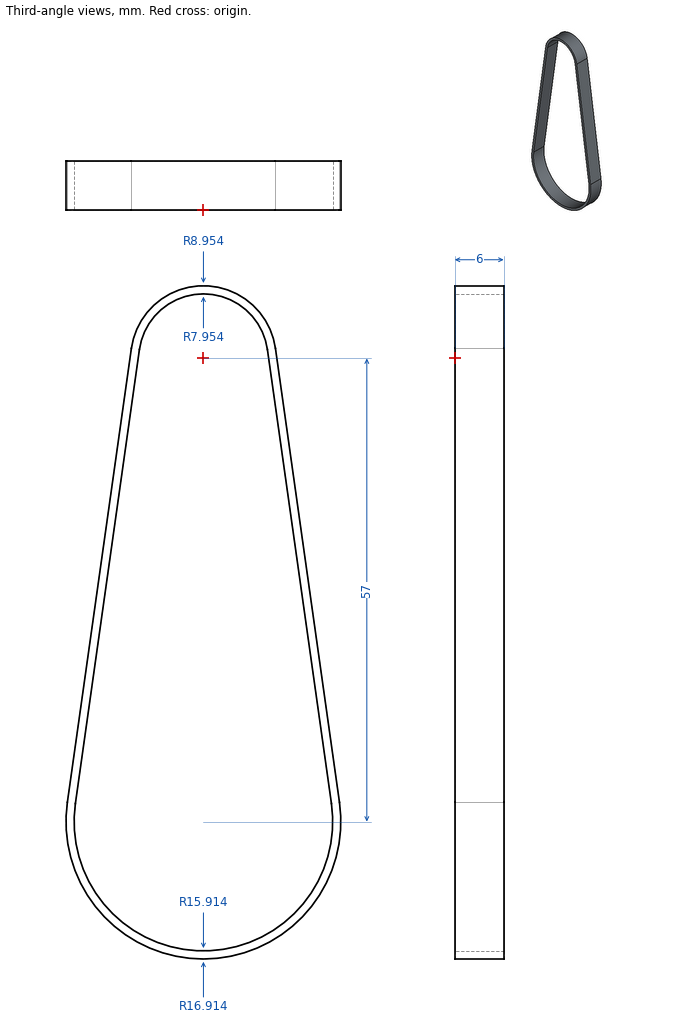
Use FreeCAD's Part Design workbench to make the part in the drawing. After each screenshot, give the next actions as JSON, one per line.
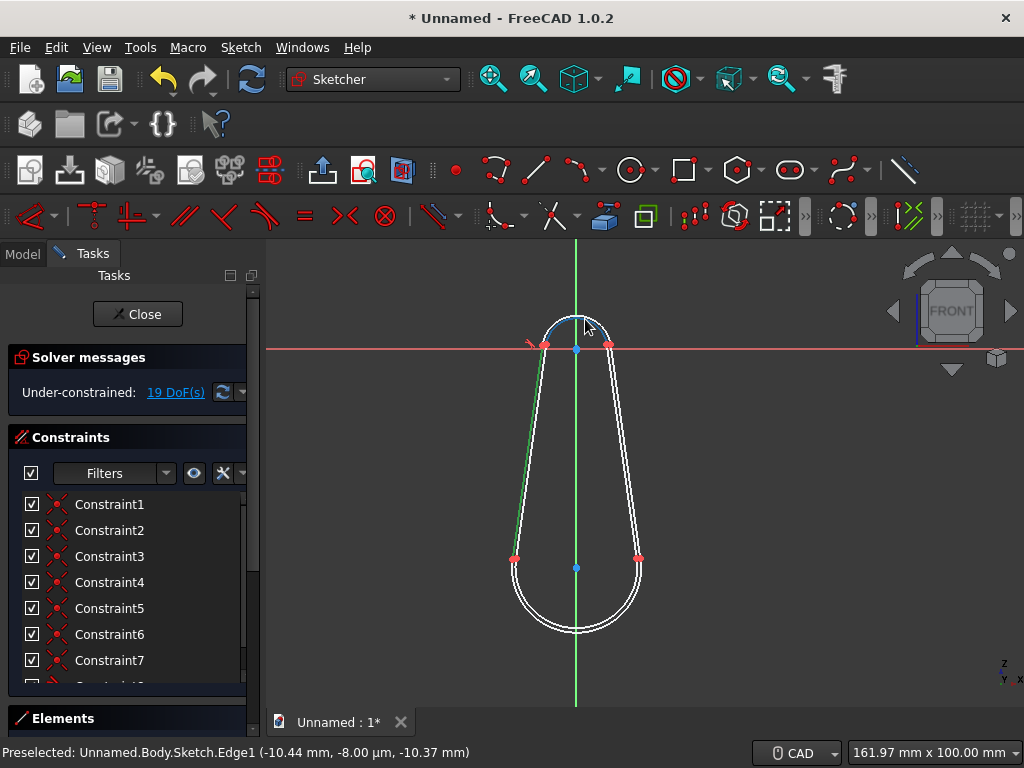
{"action": "scroll", "coordinate": [536, 618], "scroll_direction": "up", "scroll_amount": 6}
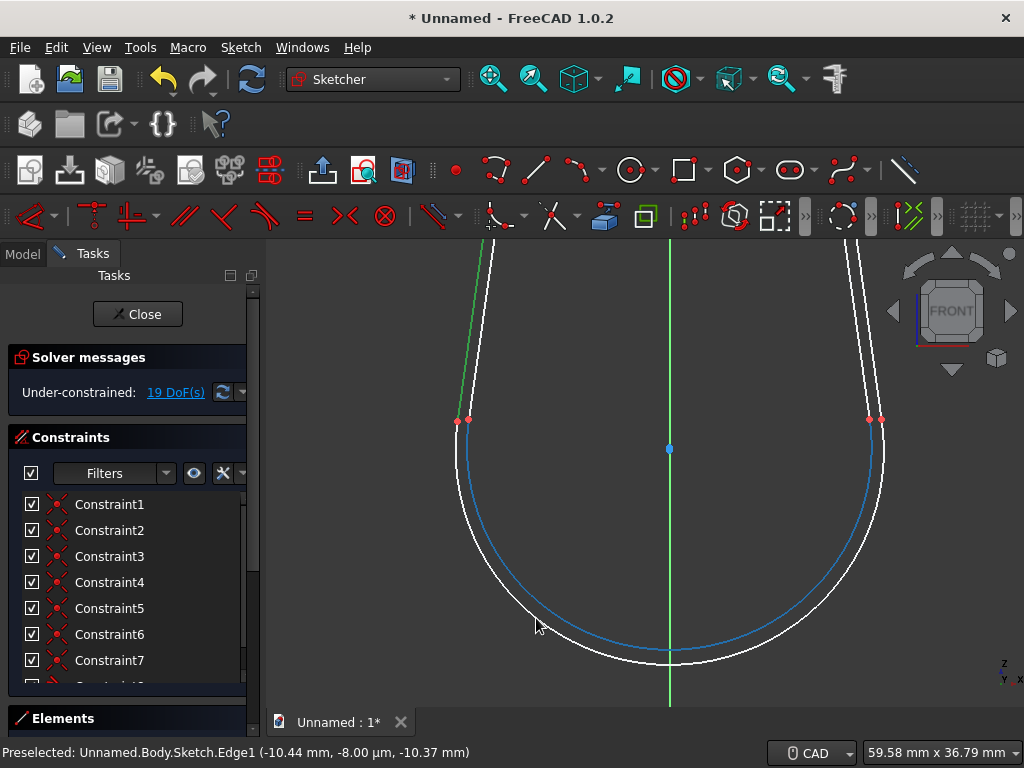
{"action": "left_click", "coordinate": [535, 617]}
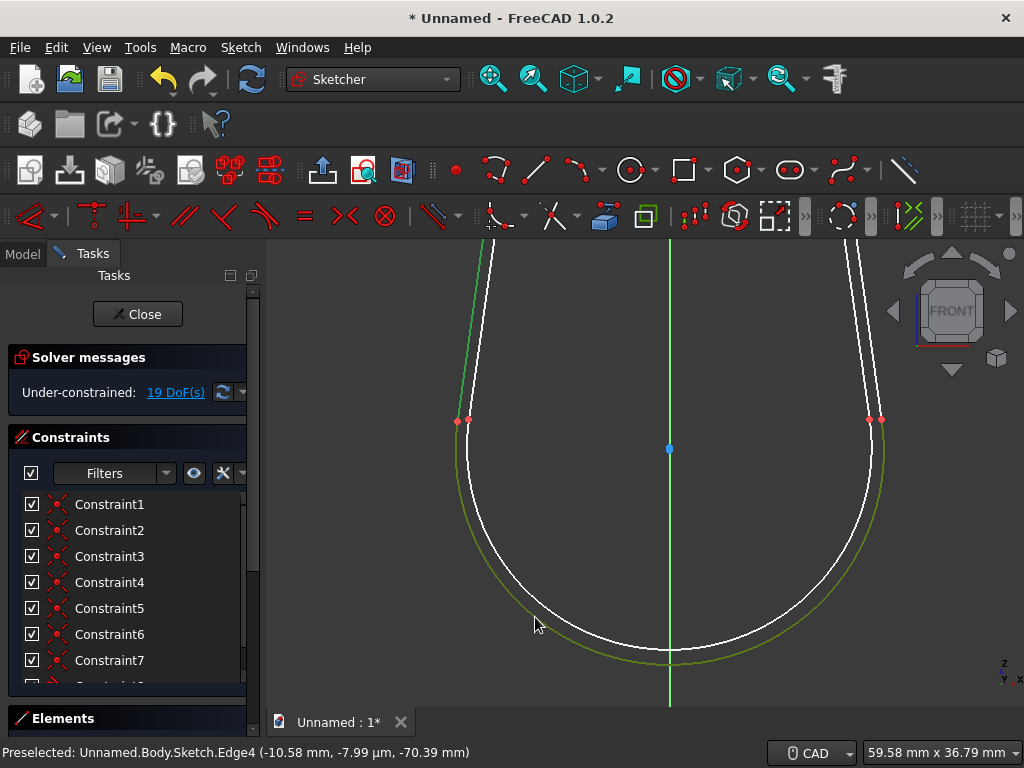
{"action": "left_click", "coordinate": [266, 216]}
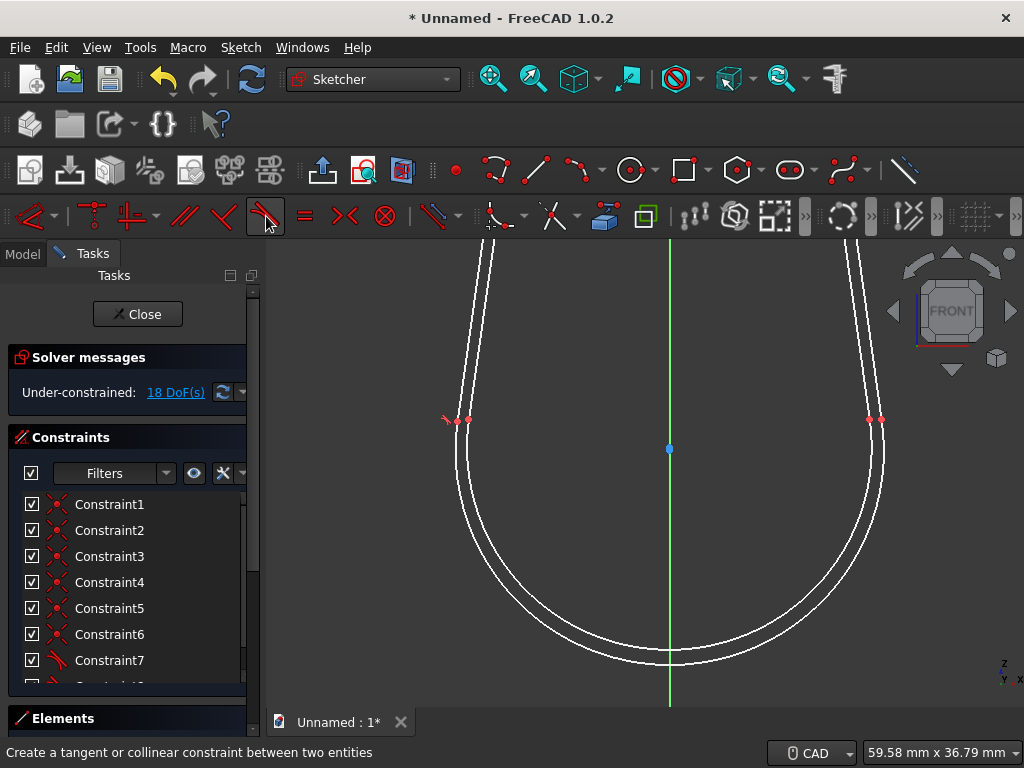
{"action": "scroll", "coordinate": [536, 619], "scroll_direction": "down", "scroll_amount": 6}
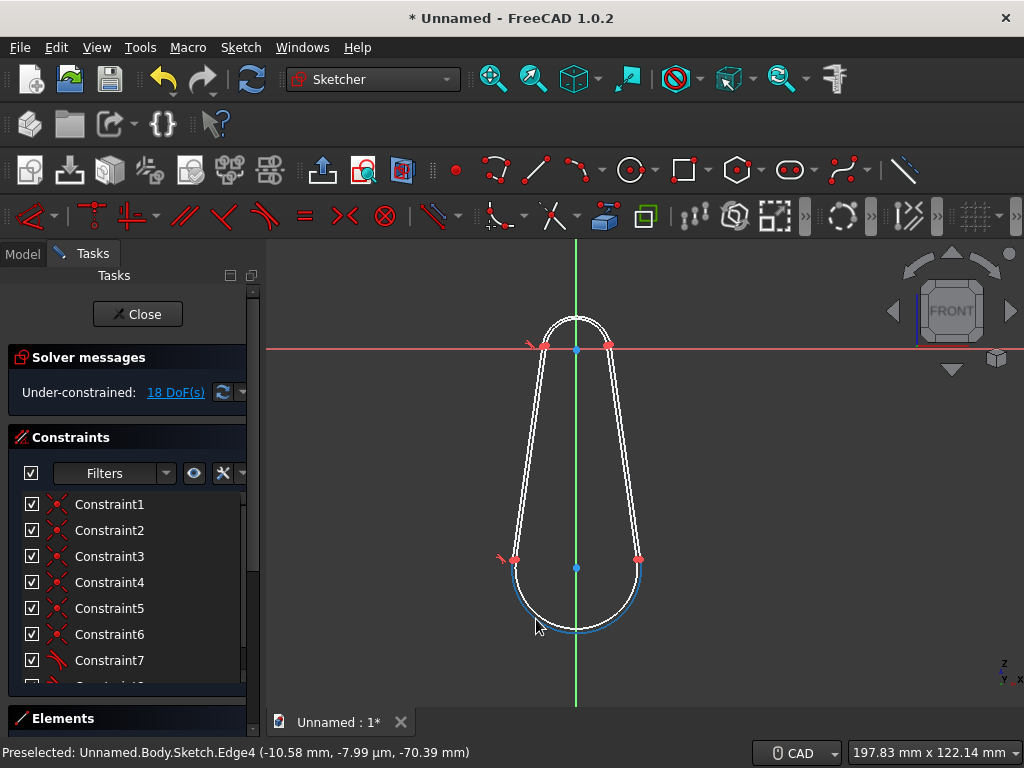
{"action": "scroll", "coordinate": [619, 409], "scroll_direction": "up", "scroll_amount": 7}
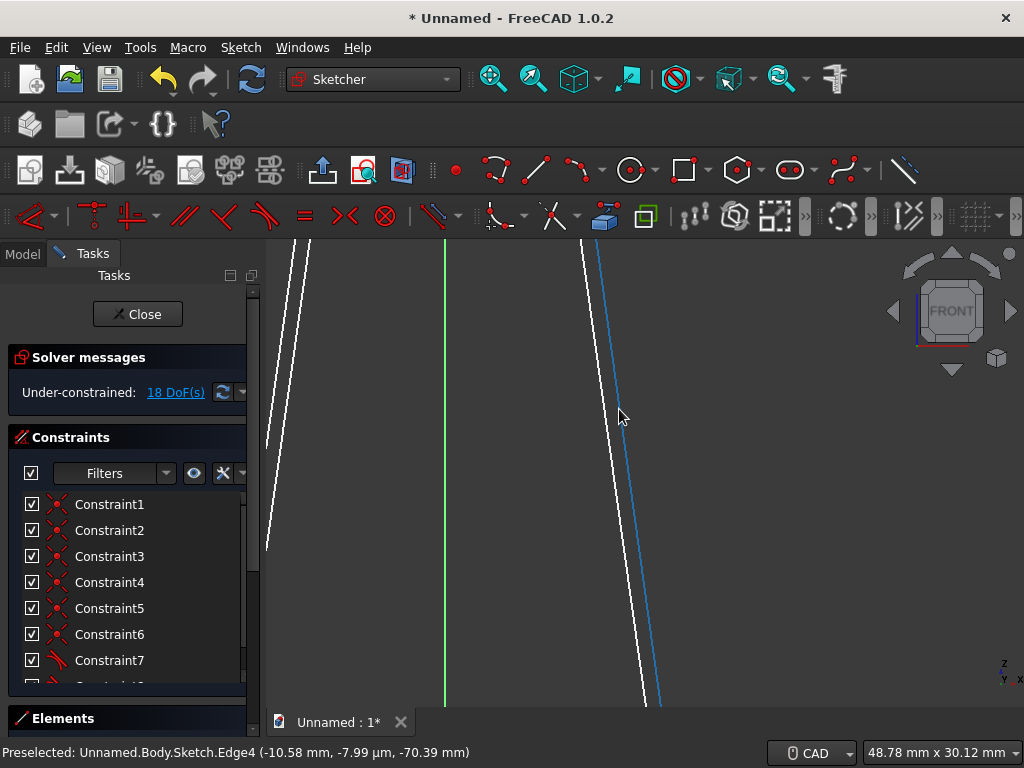
{"action": "left_click", "coordinate": [620, 408]}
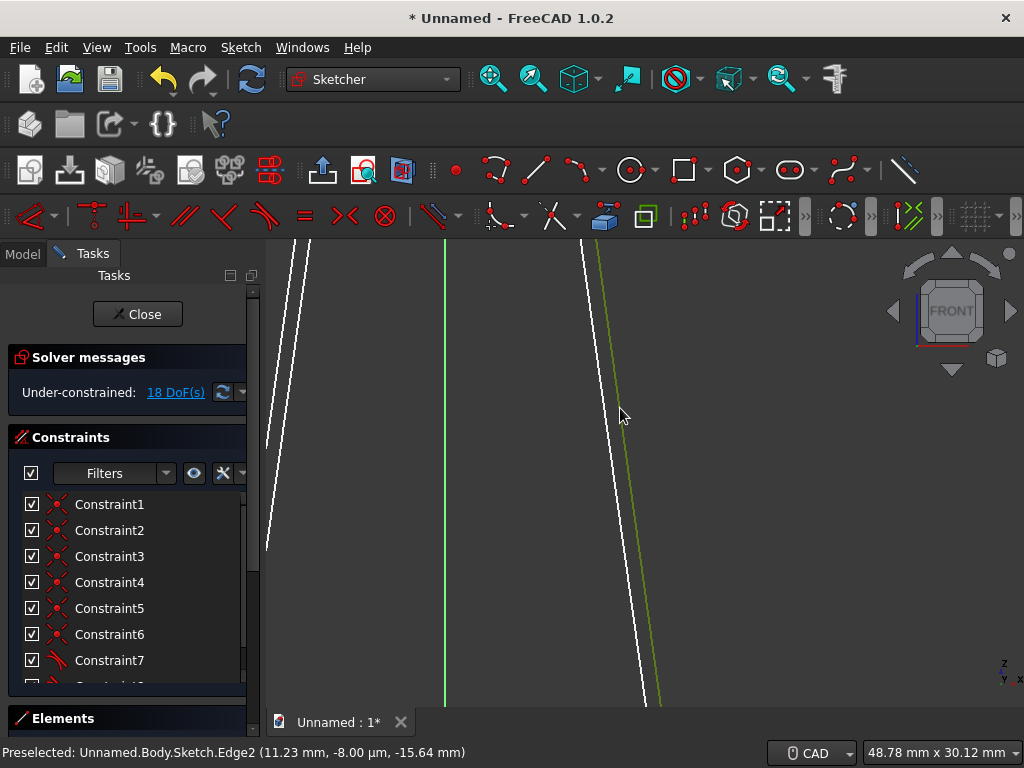
{"action": "scroll", "coordinate": [619, 408], "scroll_direction": "down", "scroll_amount": 7}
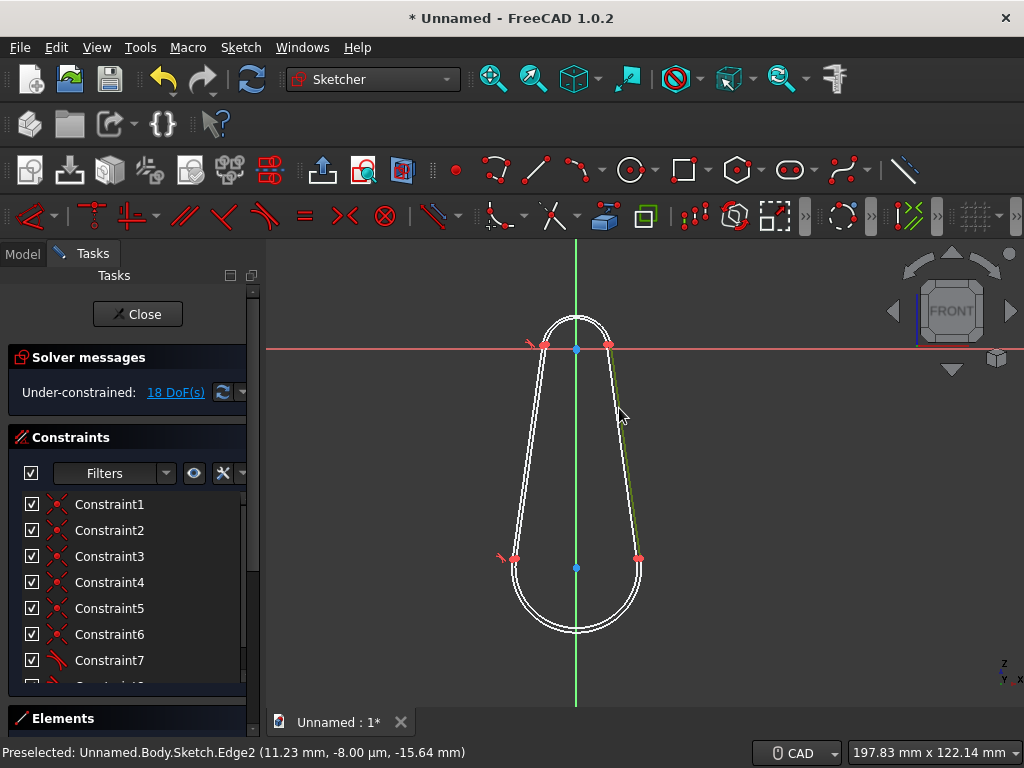
{"action": "scroll", "coordinate": [594, 321], "scroll_direction": "up", "scroll_amount": 8}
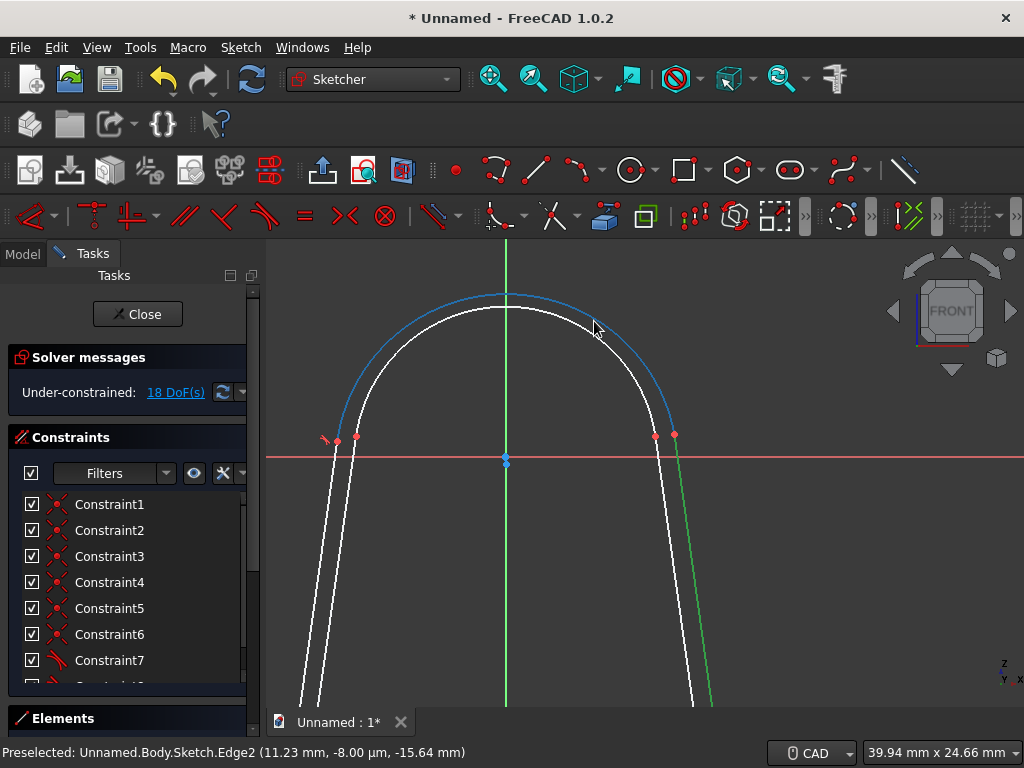
{"action": "left_click", "coordinate": [595, 319]}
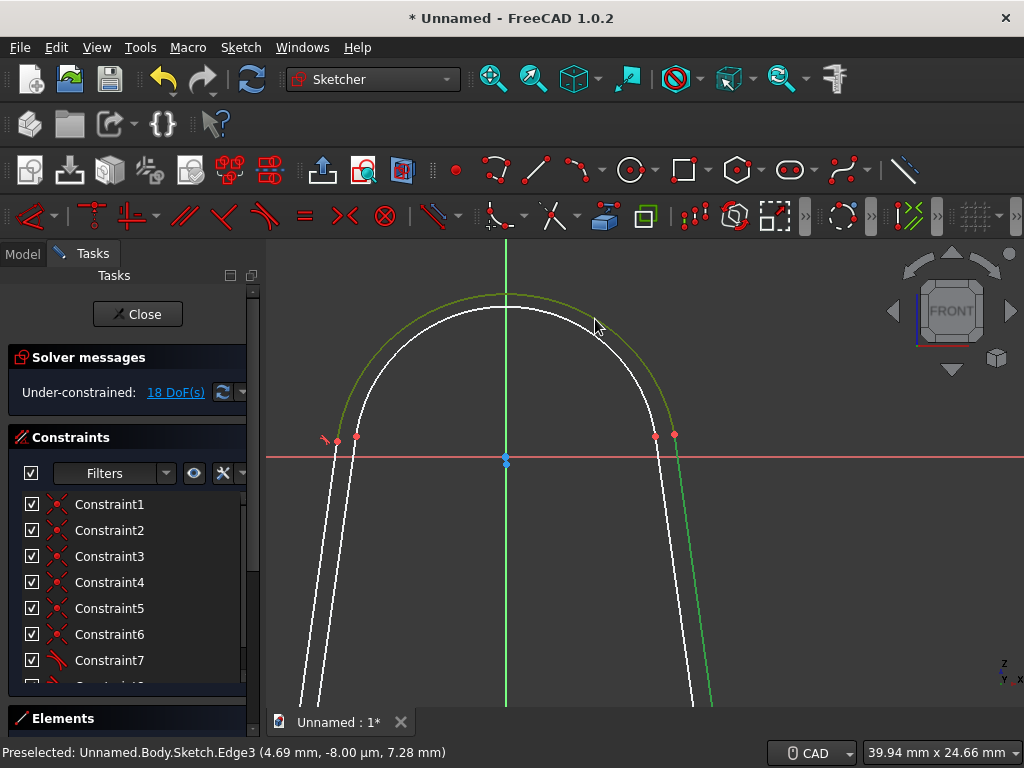
{"action": "left_click", "coordinate": [266, 216]}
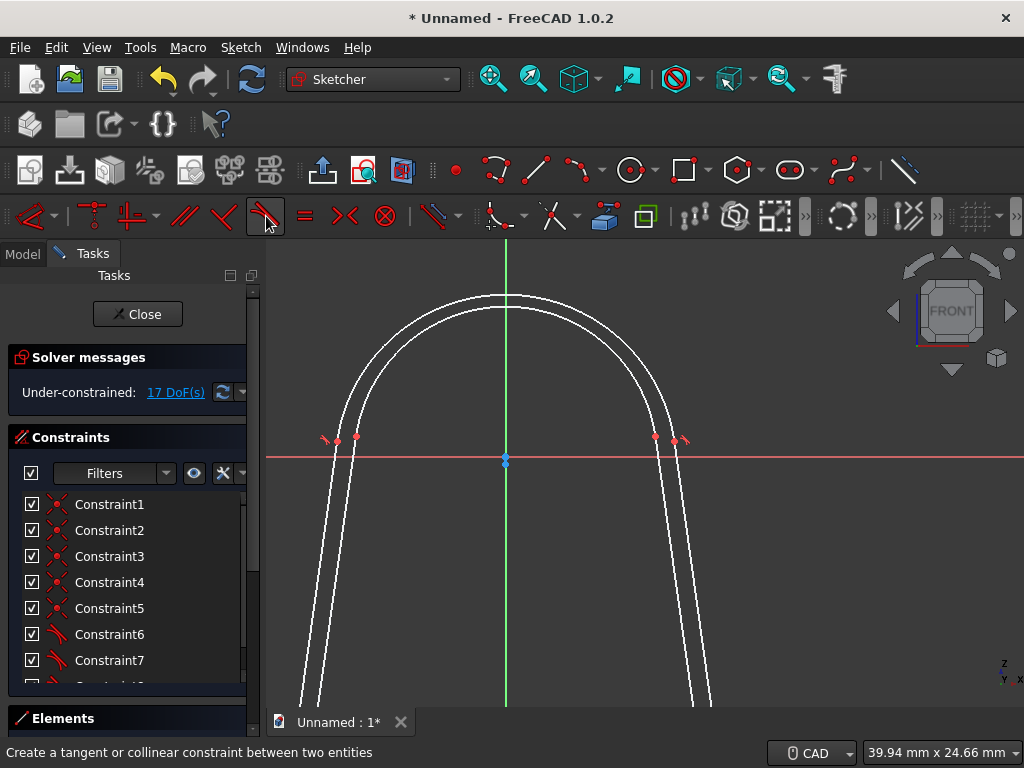
{"action": "left_click", "coordinate": [704, 653]}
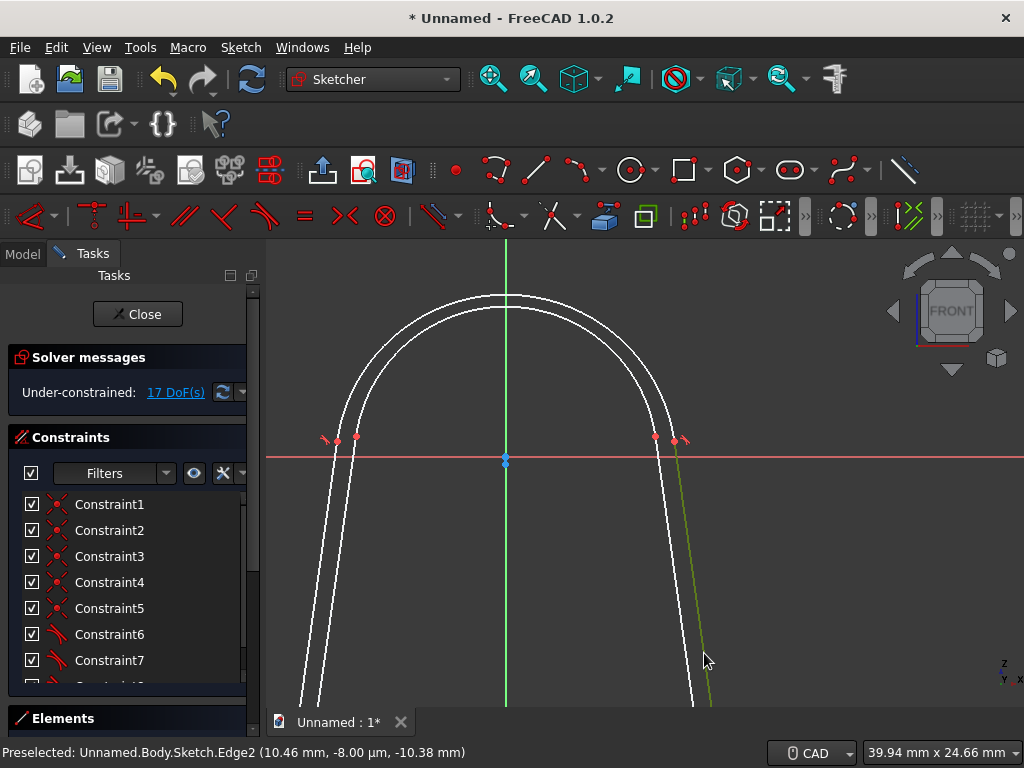
{"action": "scroll", "coordinate": [594, 321], "scroll_direction": "down", "scroll_amount": 8}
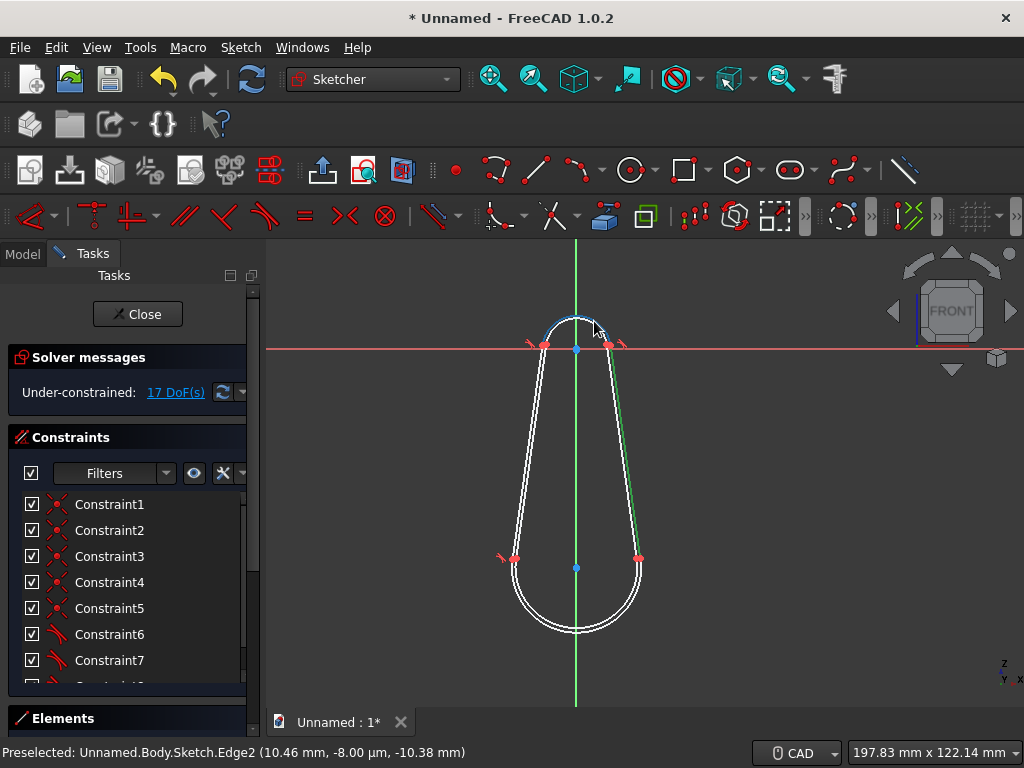
{"action": "scroll", "coordinate": [536, 618], "scroll_direction": "up", "scroll_amount": 6}